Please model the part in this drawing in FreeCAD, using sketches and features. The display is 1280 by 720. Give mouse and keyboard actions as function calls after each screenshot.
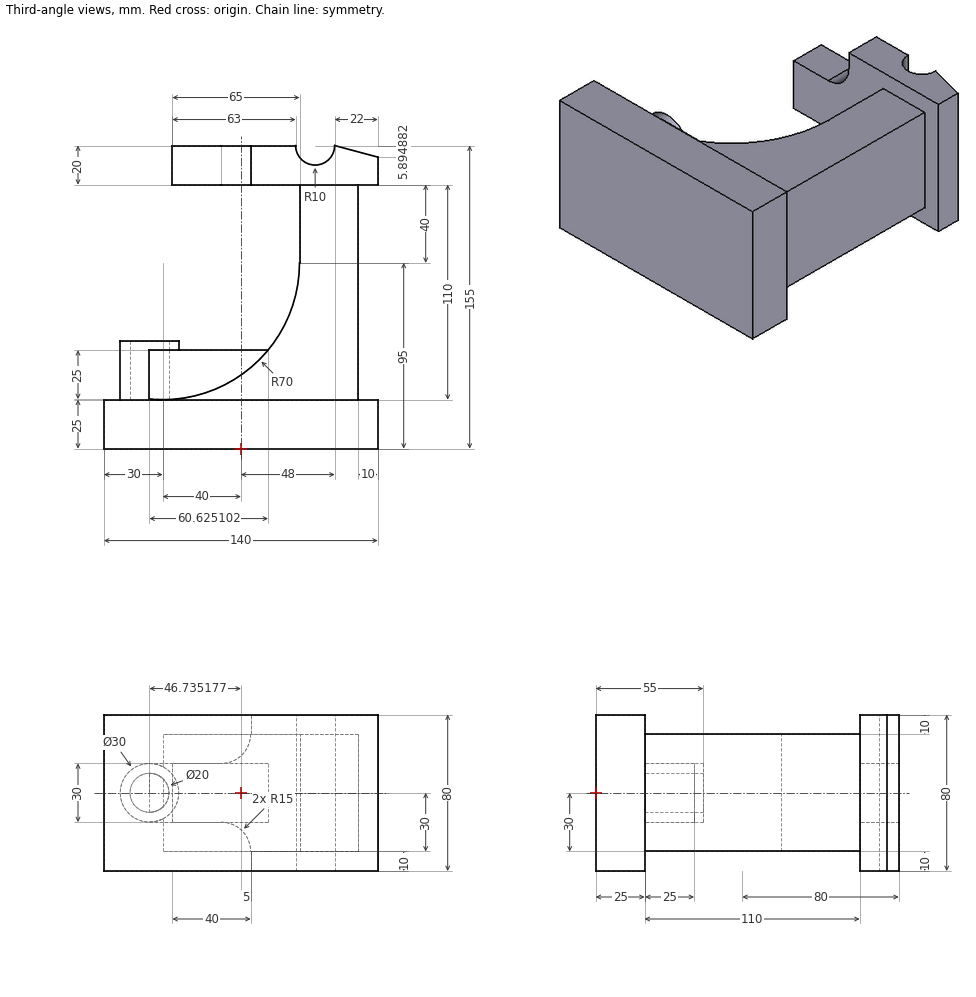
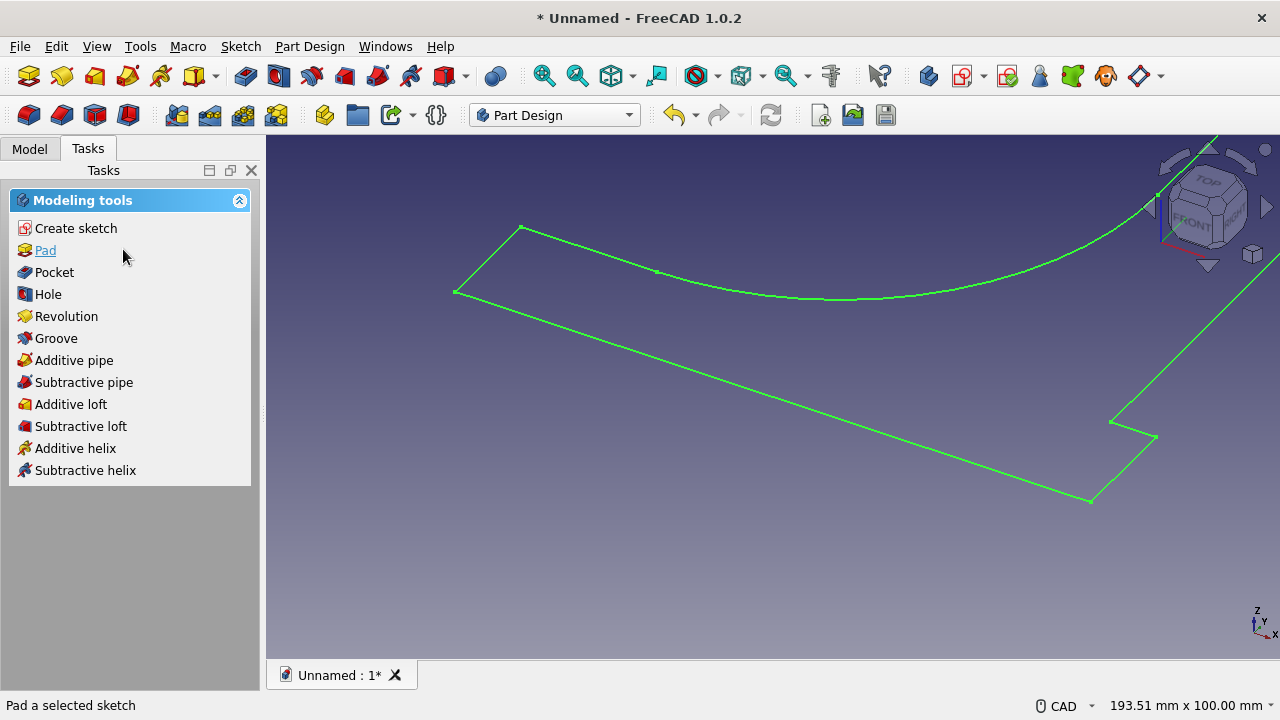
click(29, 76)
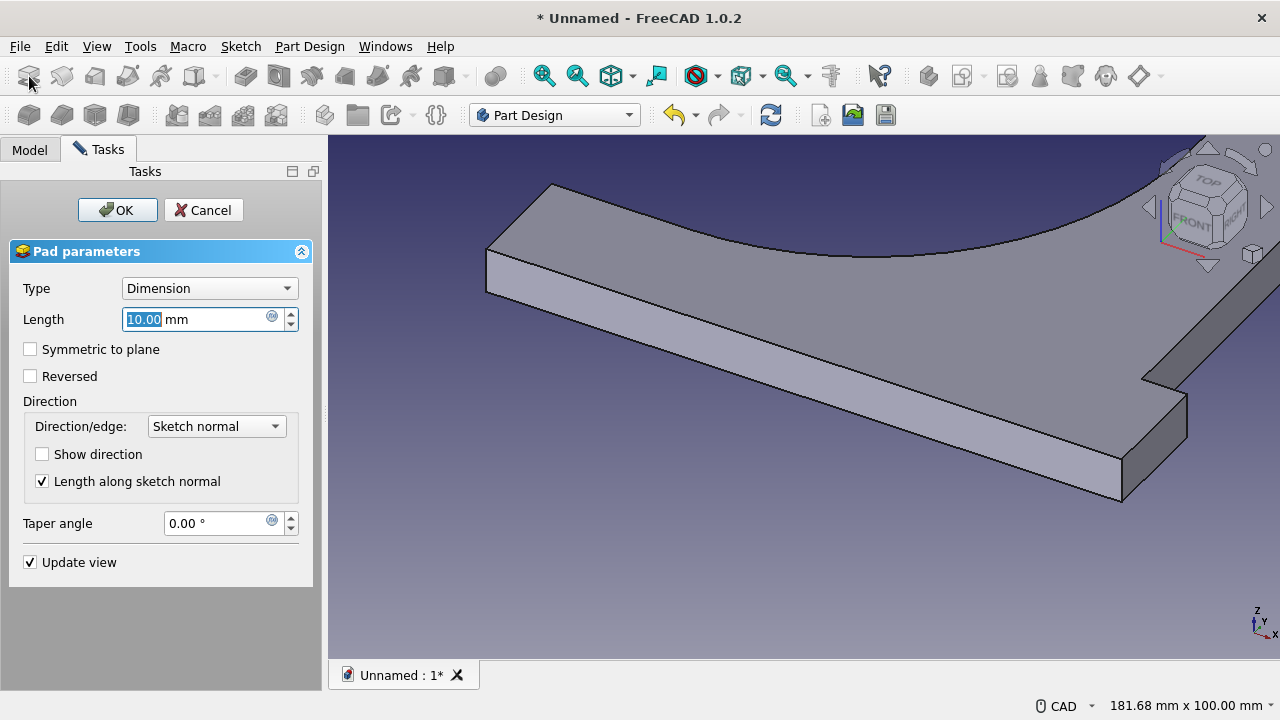
text(80)
key(Tab)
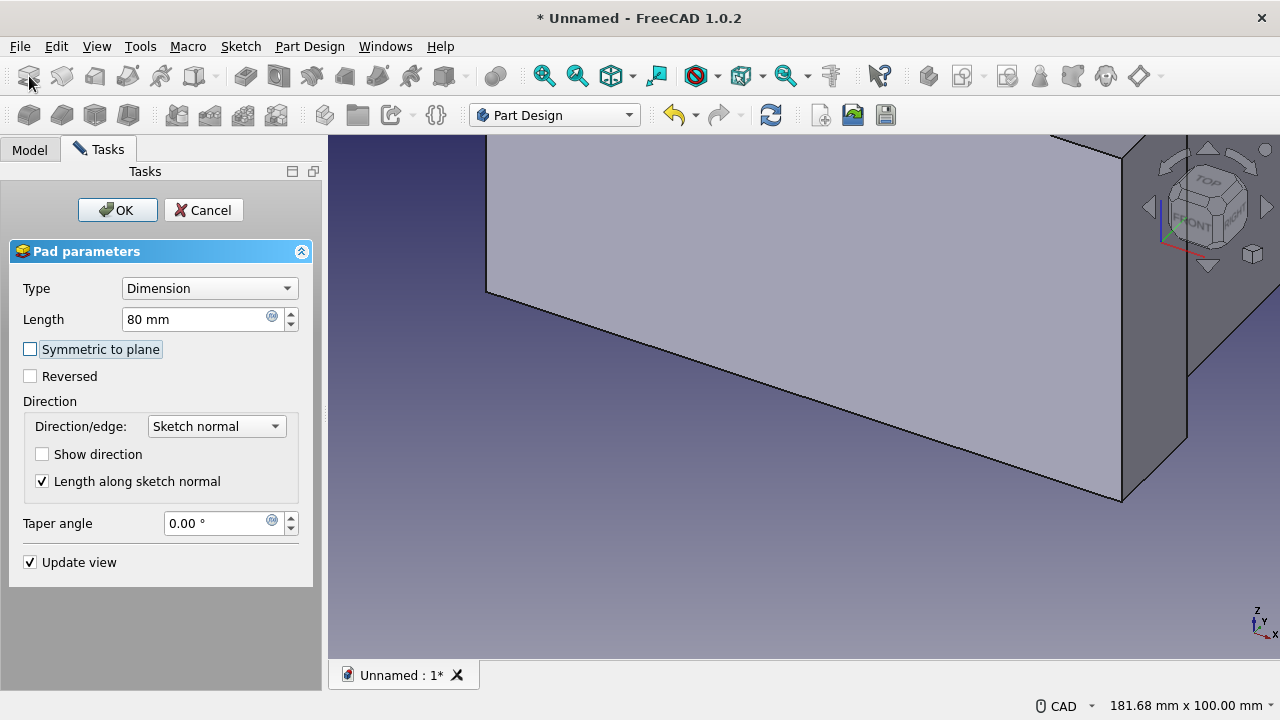
click(31, 349)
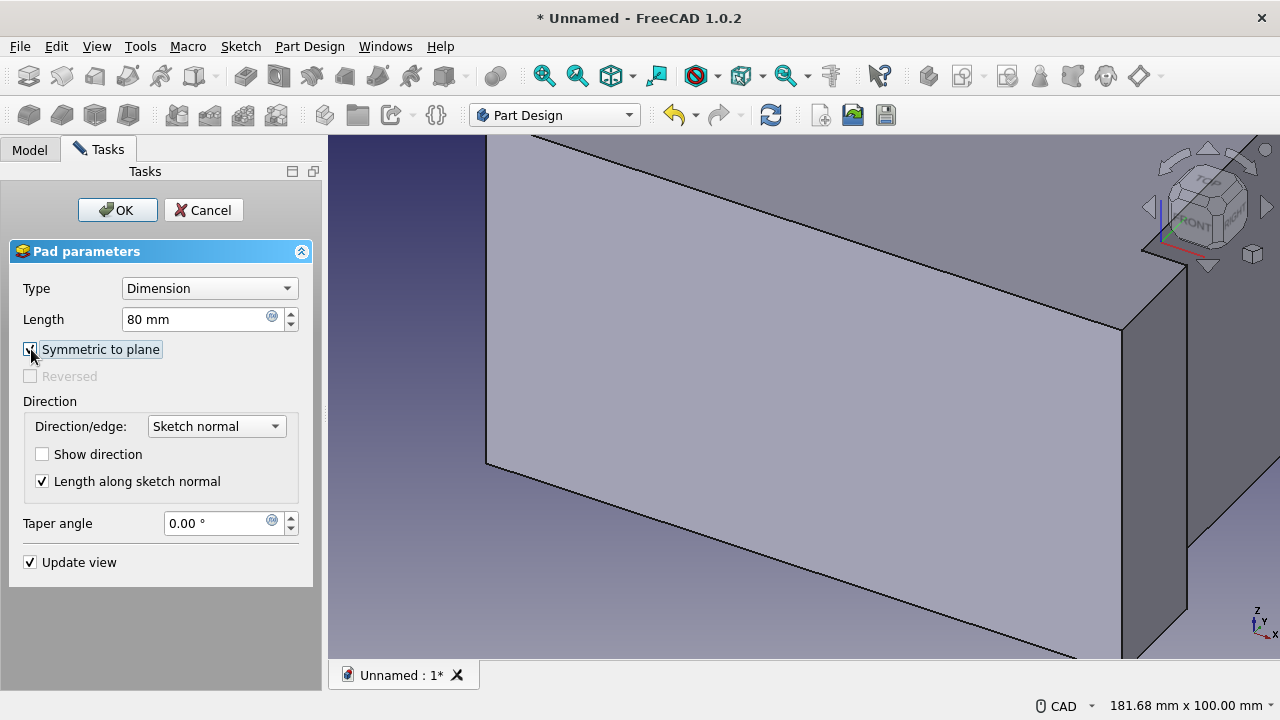
click(118, 210)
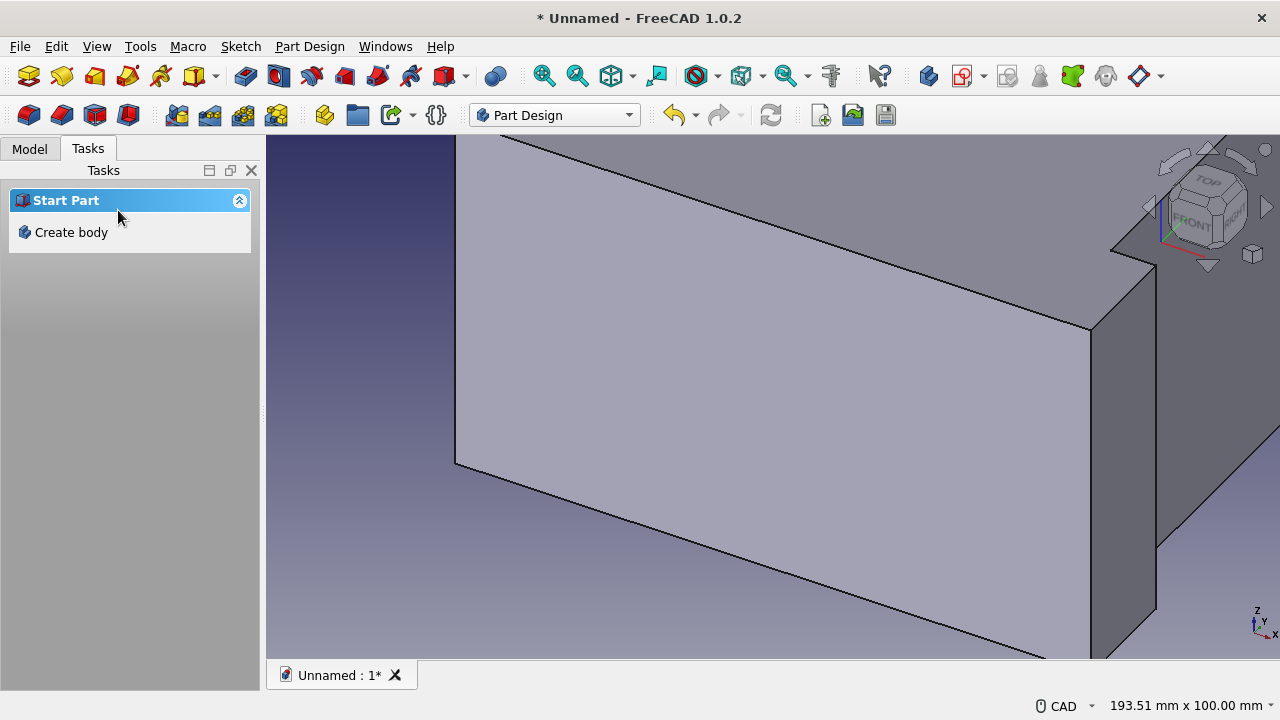
click(545, 76)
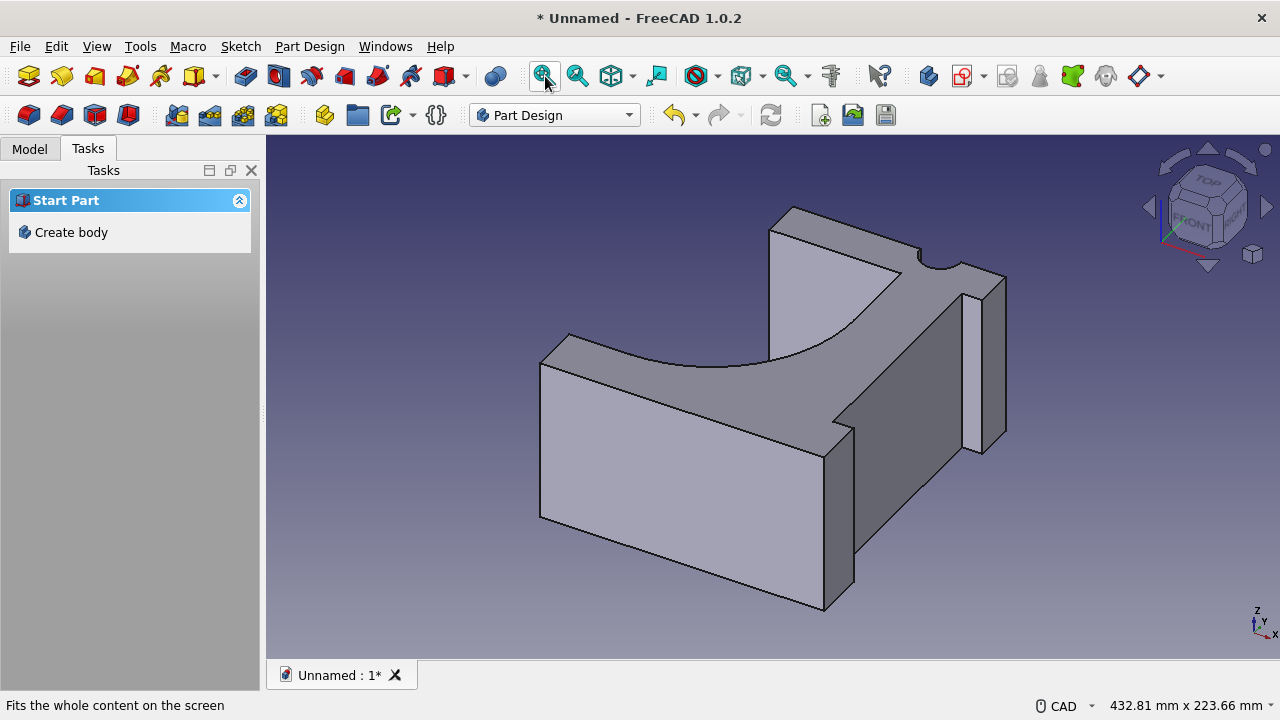
click(898, 433)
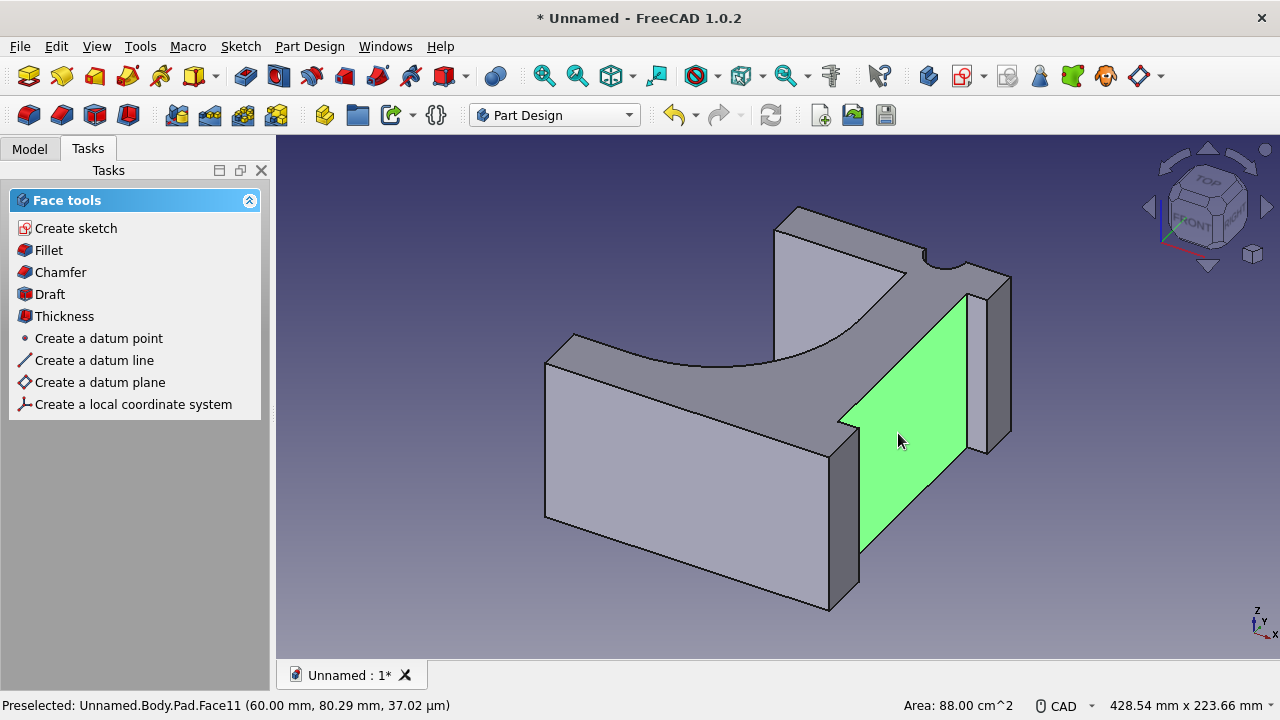
click(962, 76)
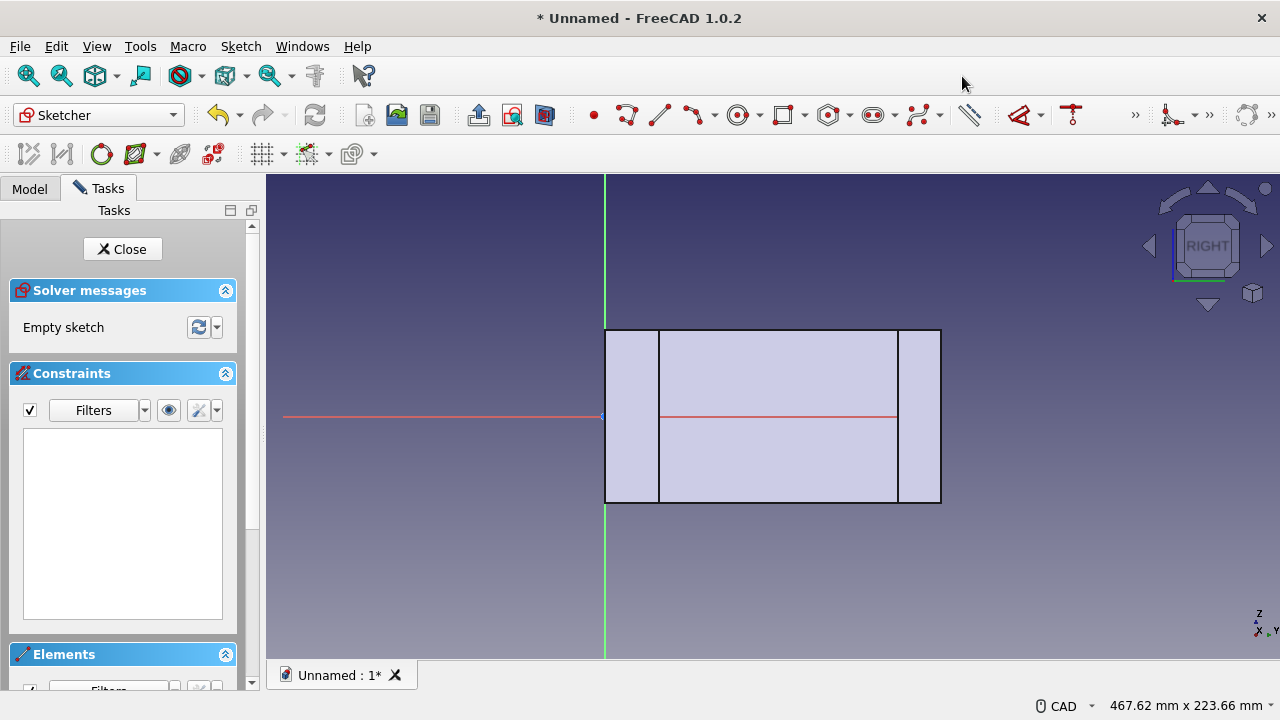
scroll(808, 416, up, 3)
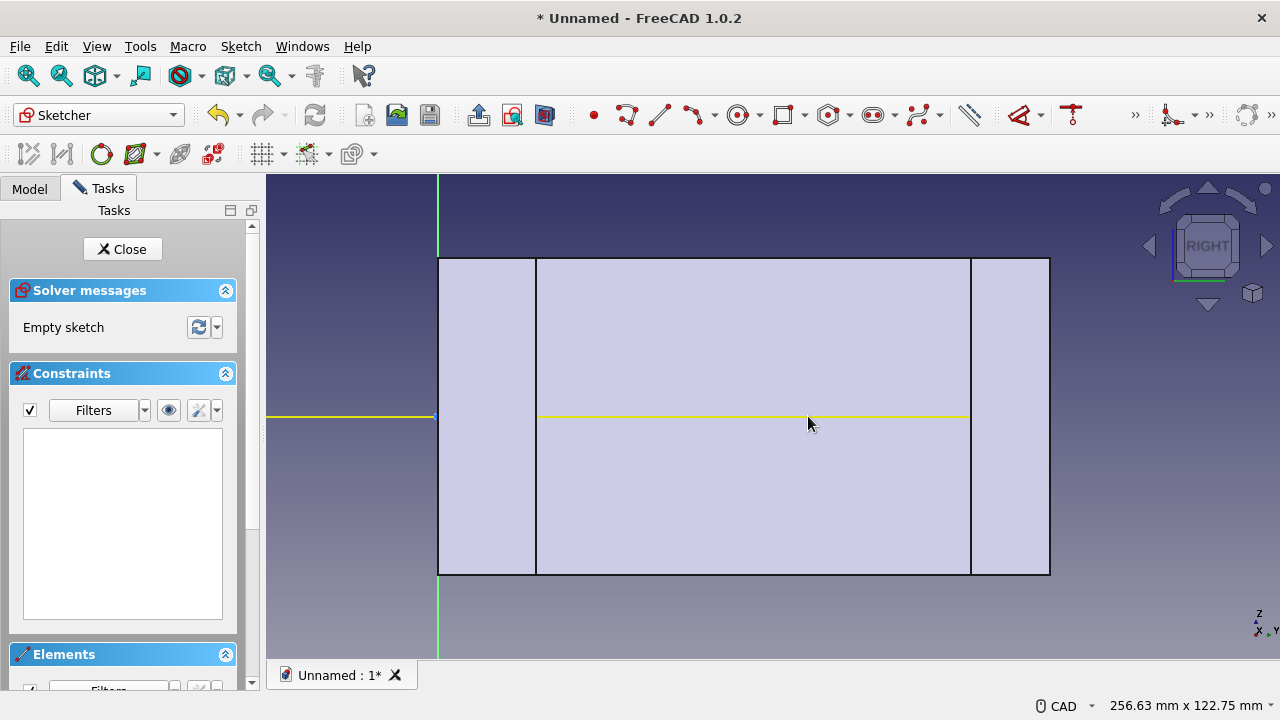
click(782, 116)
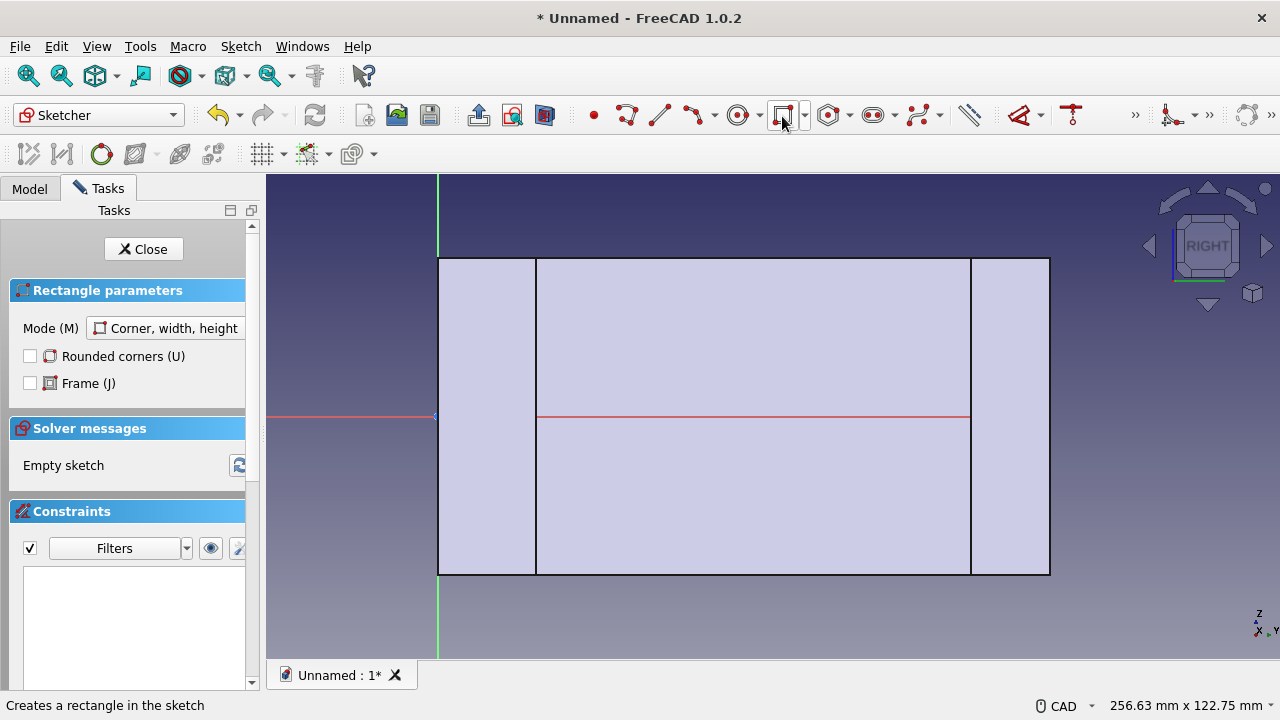
click(536, 535)
move(971, 575)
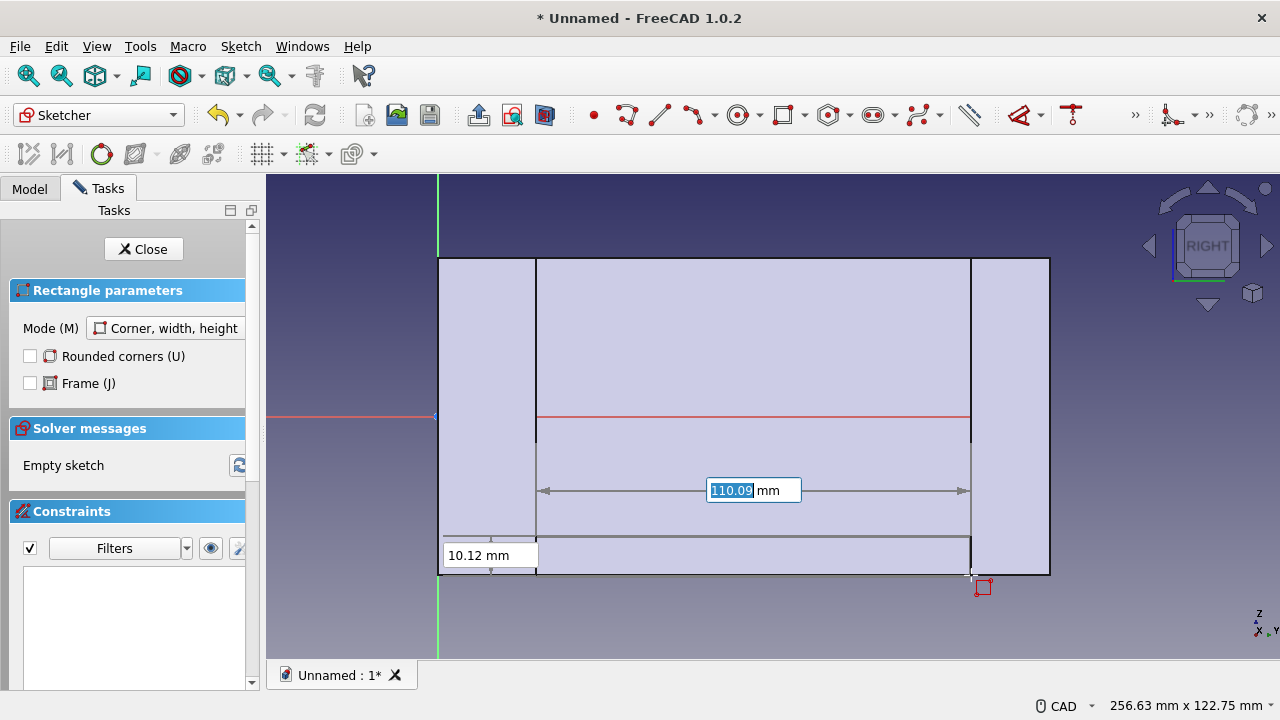
text(110)
key(Tab)
text(10)
key(Return)